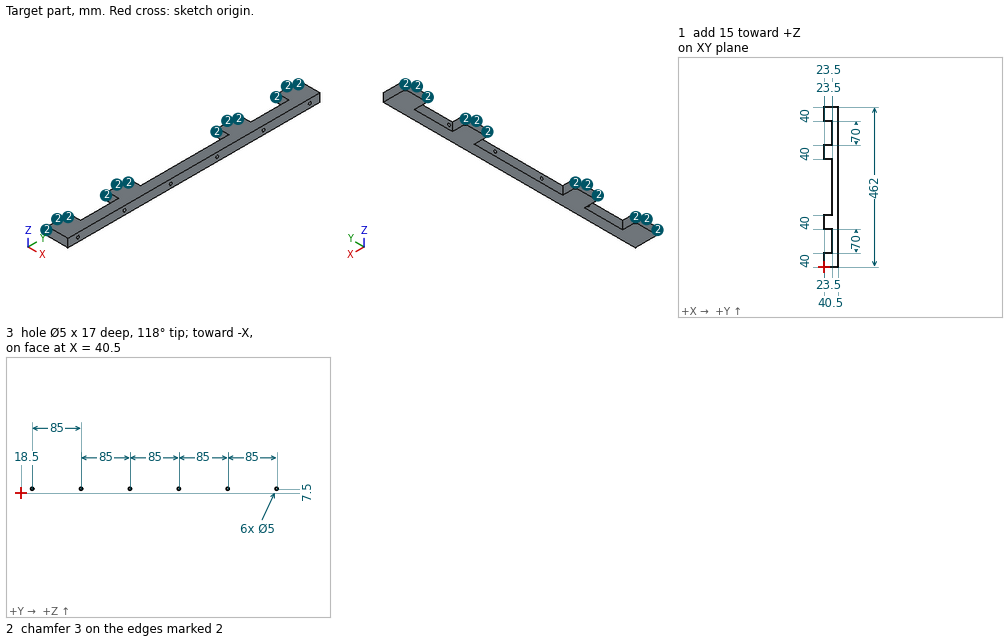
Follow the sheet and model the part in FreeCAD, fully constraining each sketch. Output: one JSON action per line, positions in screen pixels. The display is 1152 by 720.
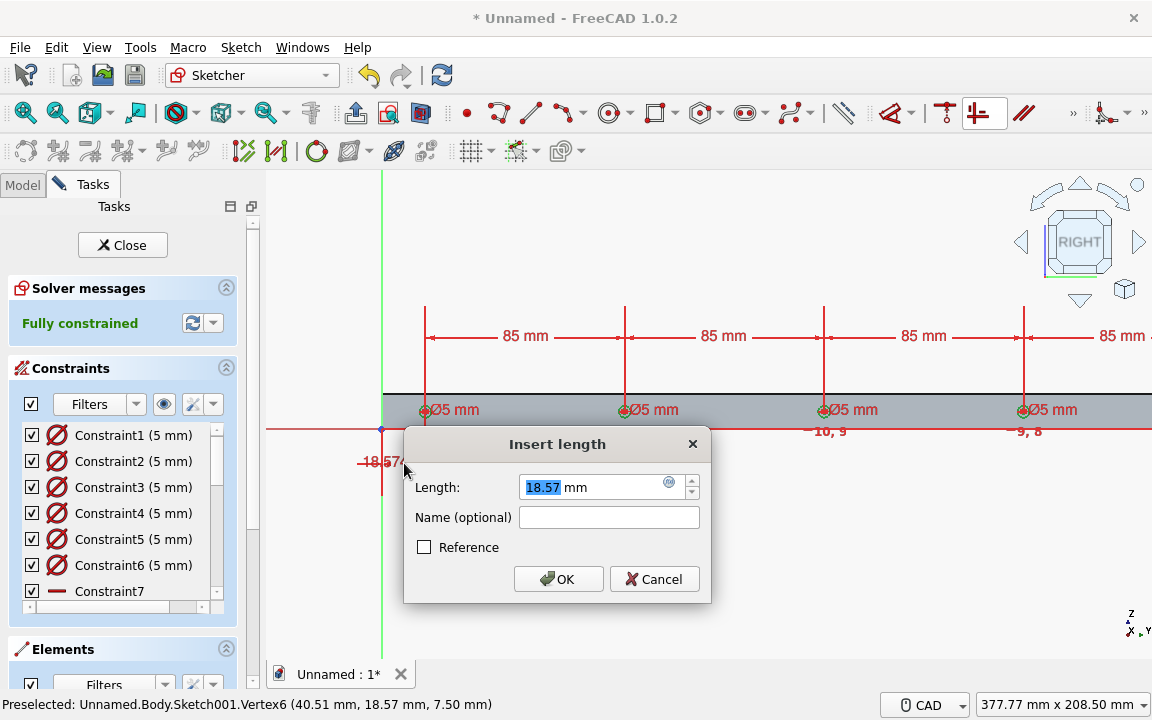
{"action": "type", "text": "18.5"}
{"action": "key", "text": "Return"}
{"action": "key", "text": "Escape"}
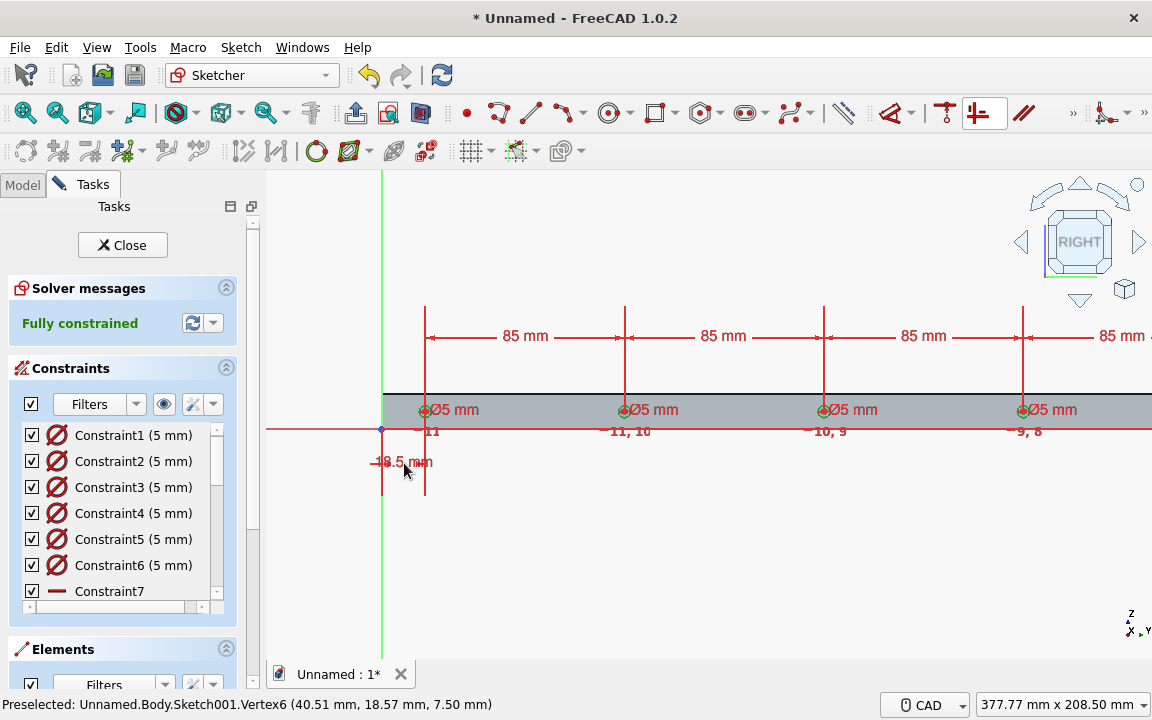
{"action": "left_click", "coordinate": [123, 245]}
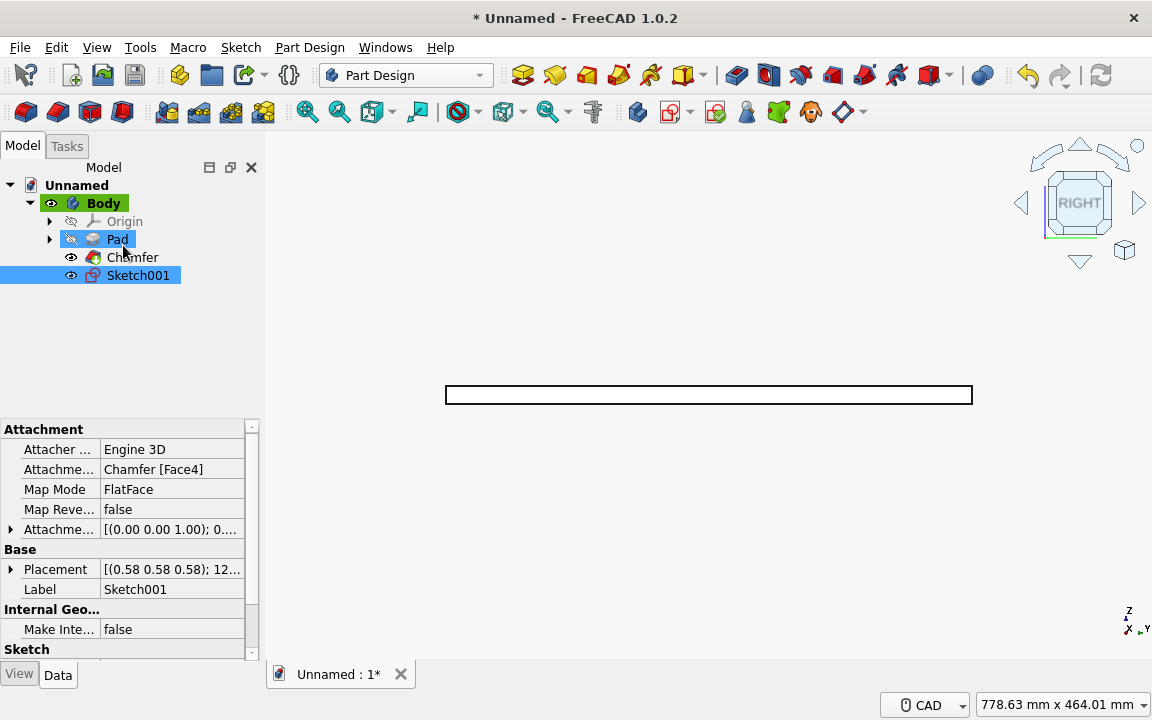
{"action": "left_click", "coordinate": [770, 76]}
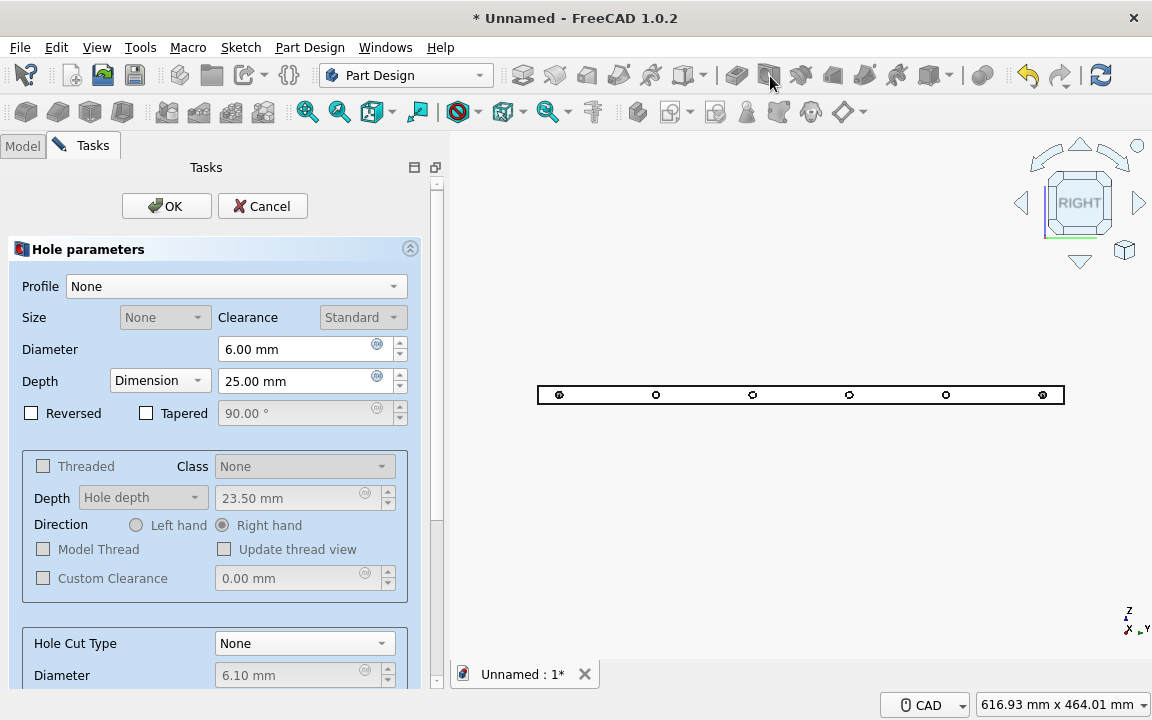
{"action": "triple_click", "coordinate": [305, 349]}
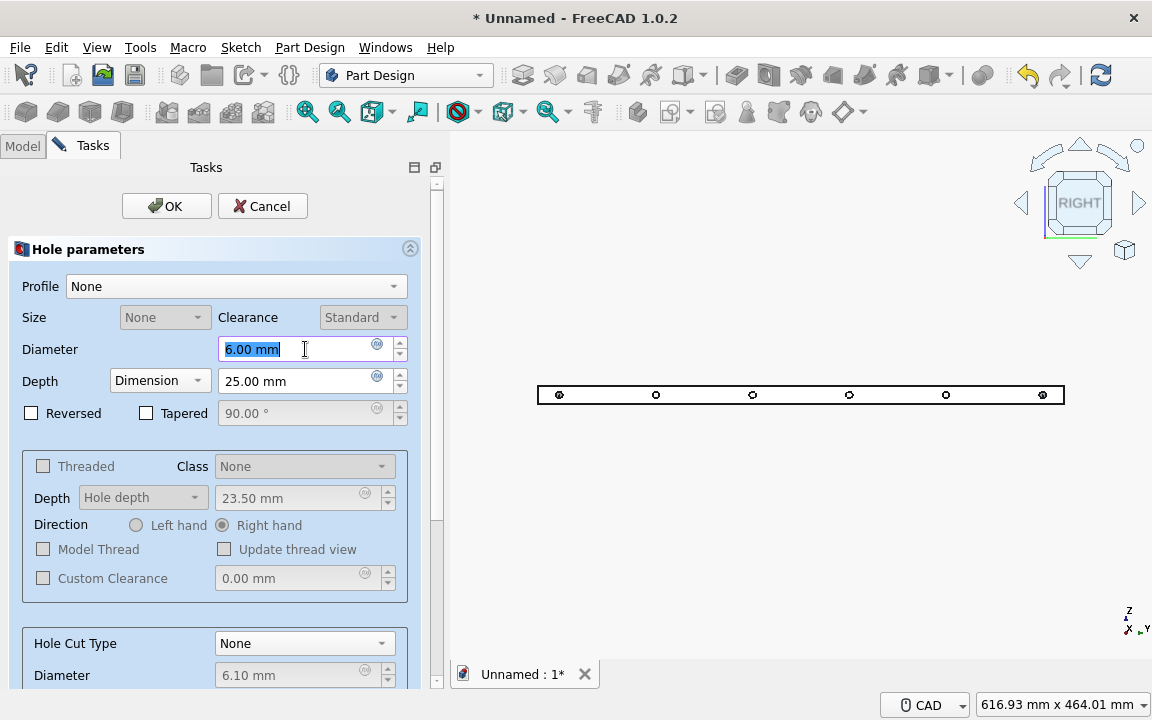
{"action": "type", "text": "5"}
{"action": "key", "text": "Tab"}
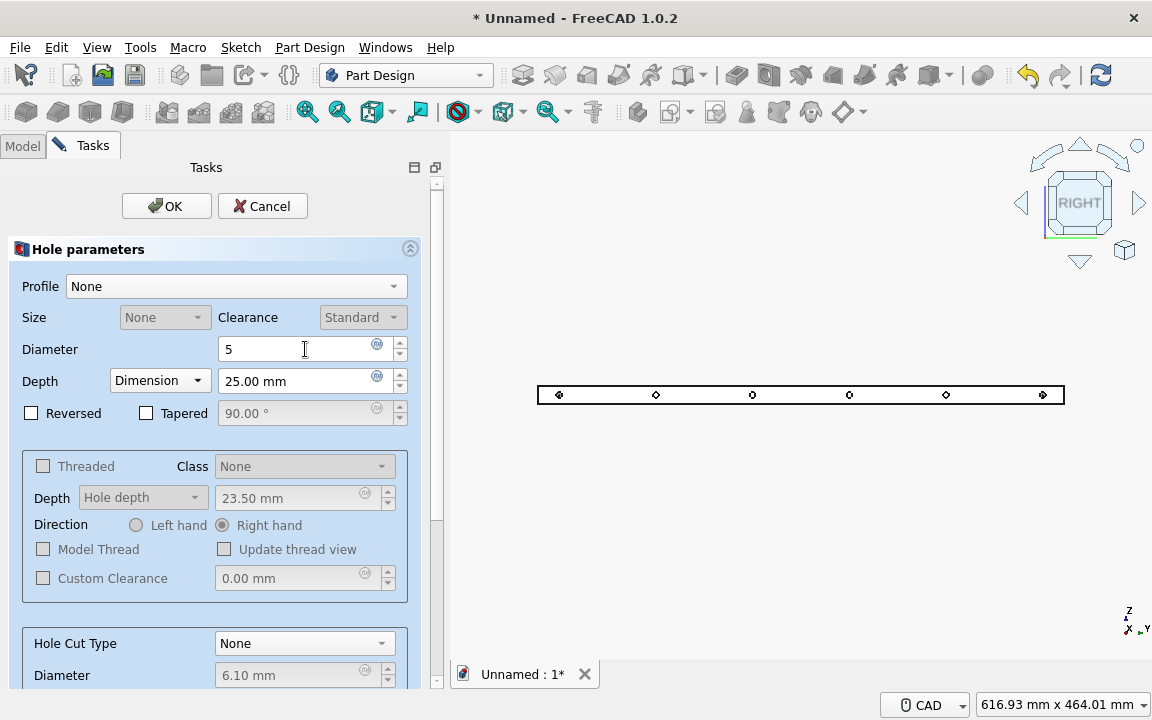
{"action": "triple_click", "coordinate": [305, 381]}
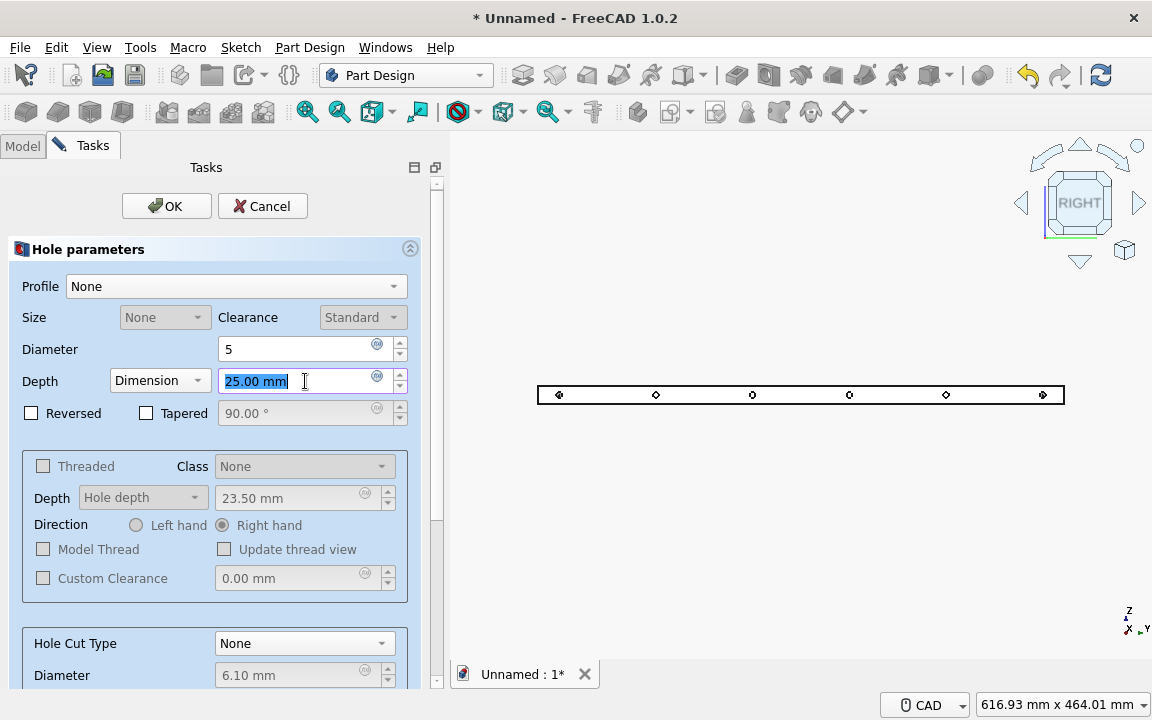
{"action": "type", "text": "17"}
{"action": "key", "text": "Tab"}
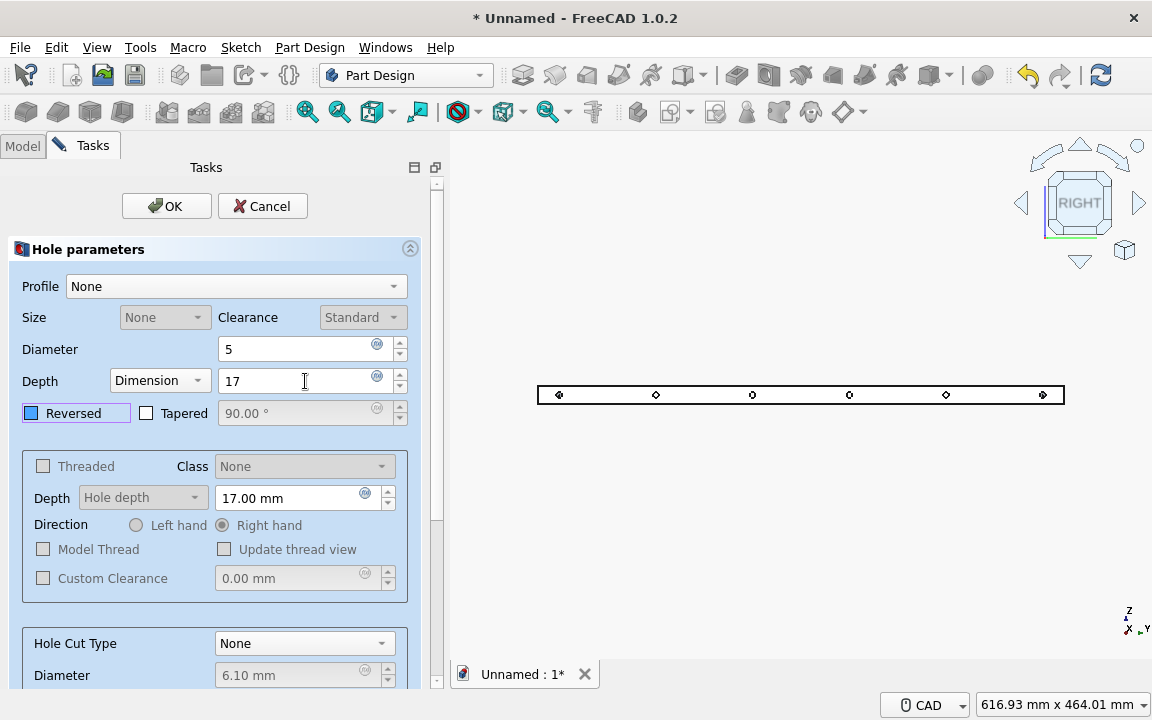
{"action": "left_click", "coordinate": [167, 206]}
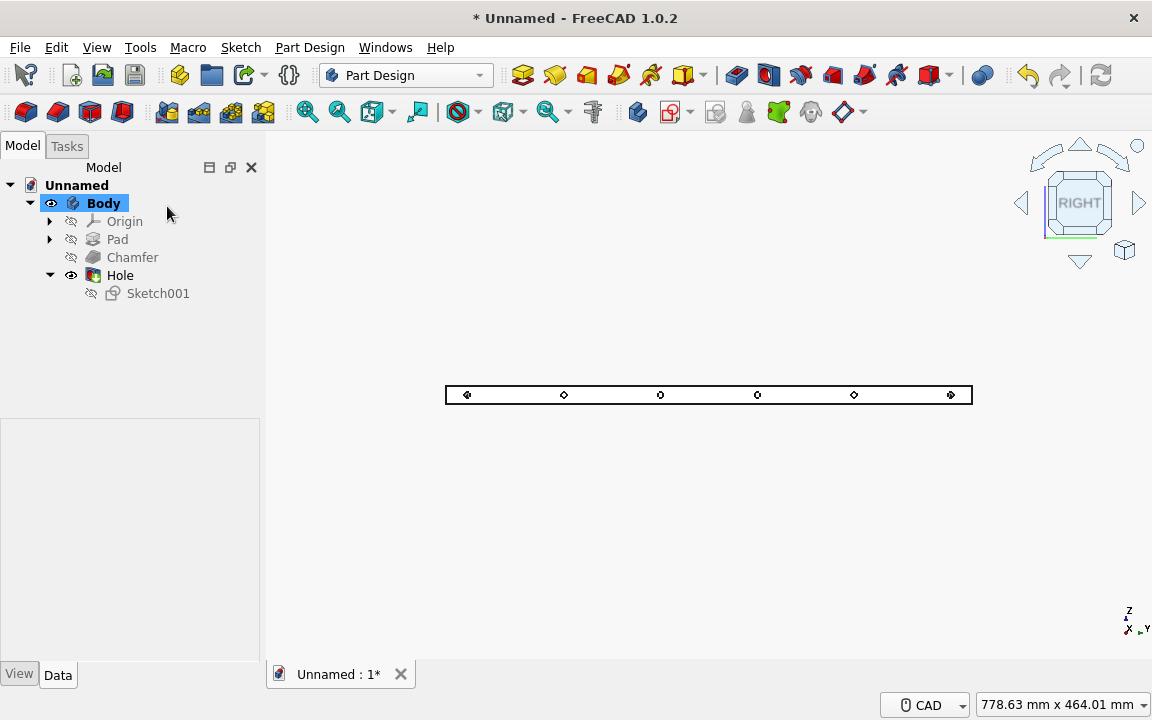
{"action": "key", "text": "0"}